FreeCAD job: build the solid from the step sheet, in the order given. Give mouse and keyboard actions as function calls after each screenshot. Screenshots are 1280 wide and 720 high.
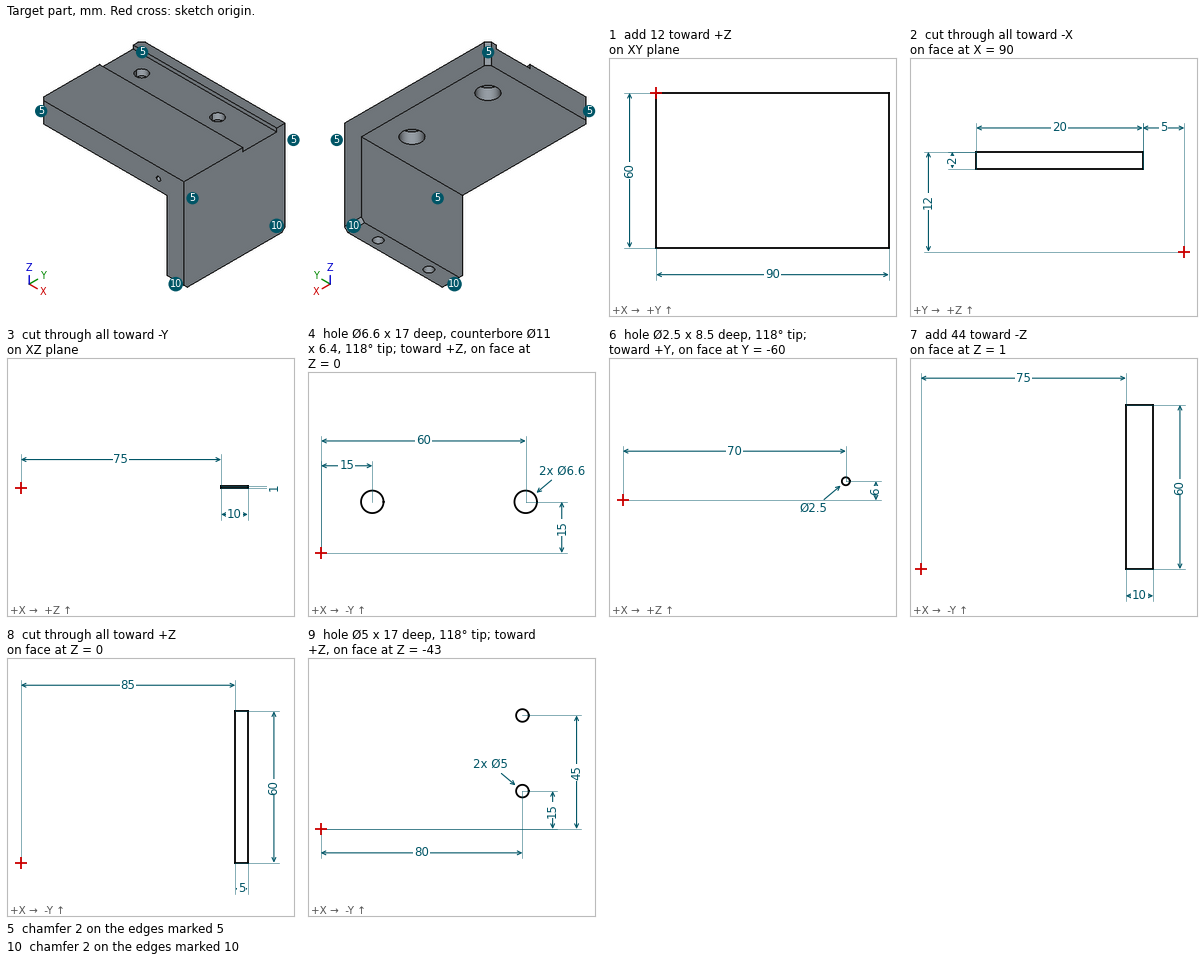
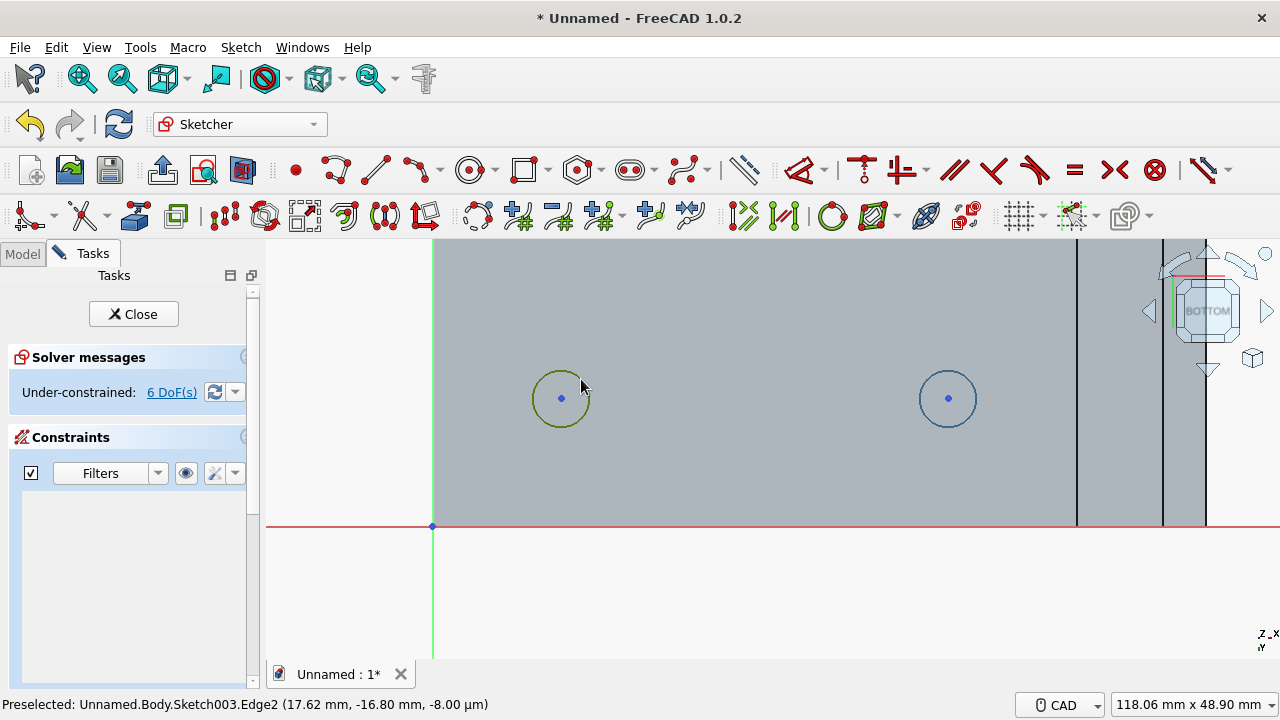
key(e)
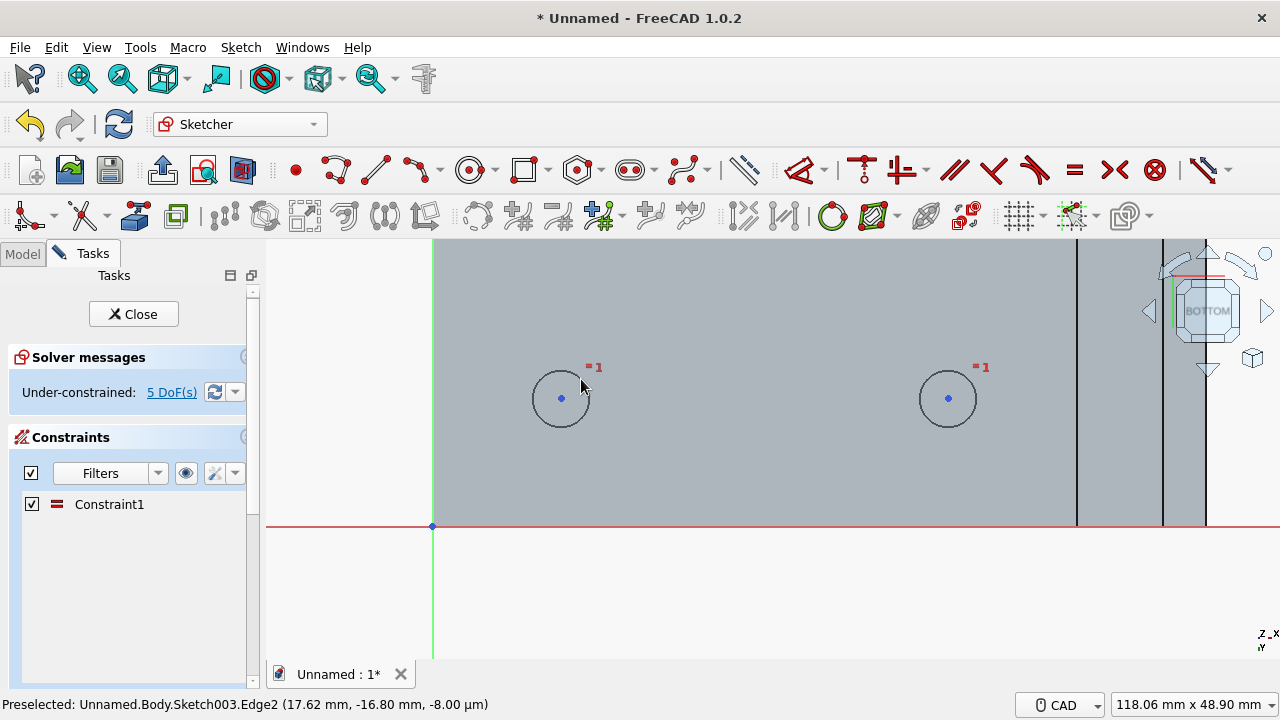
click(948, 399)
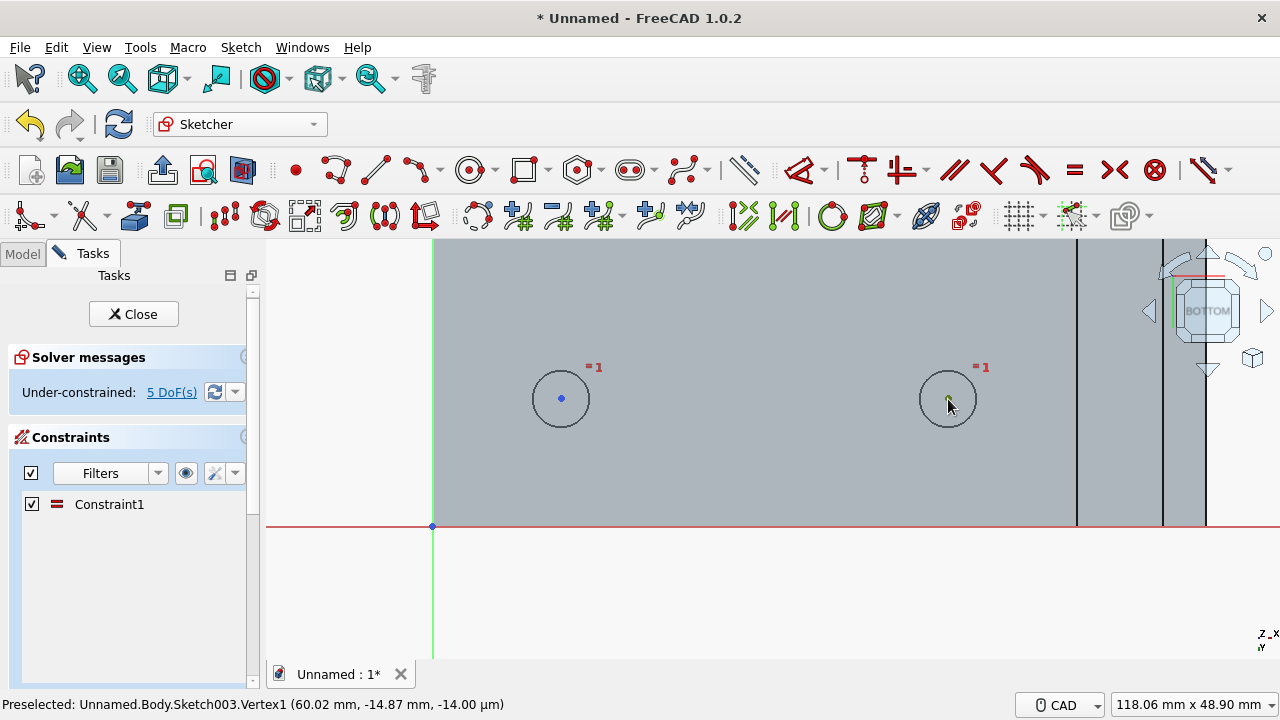
click(561, 399)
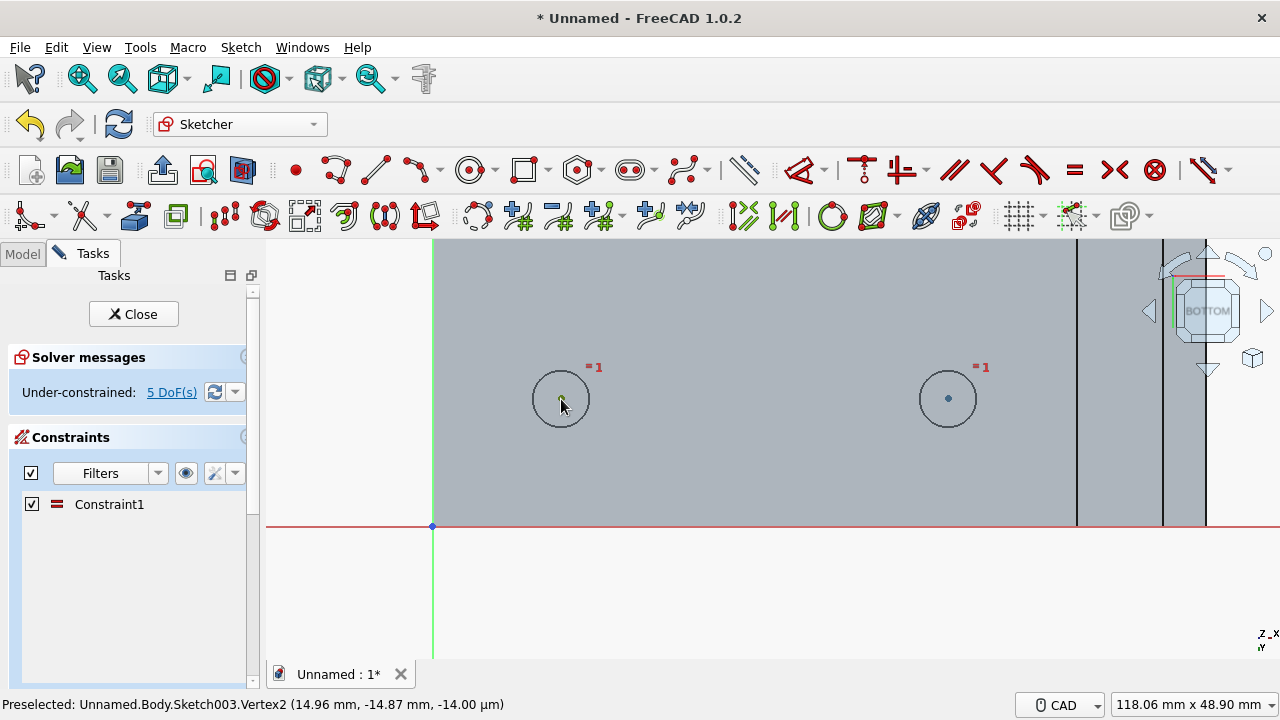
key(h)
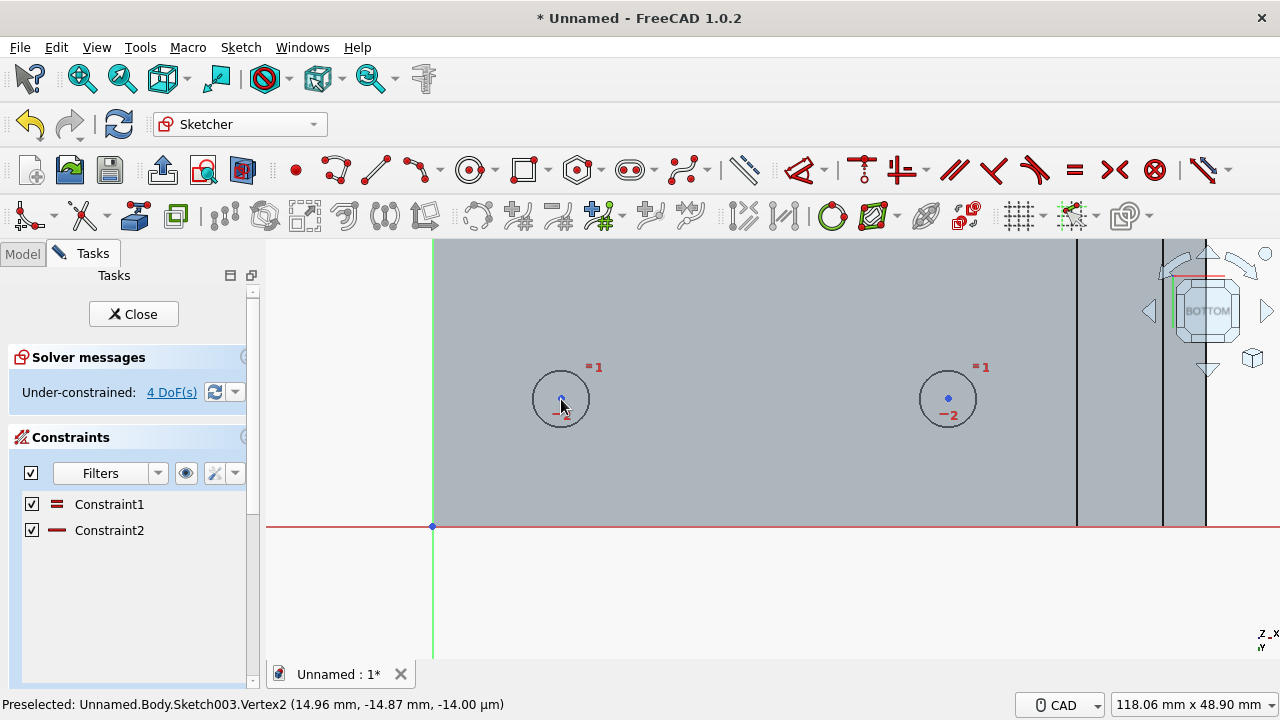
key(d)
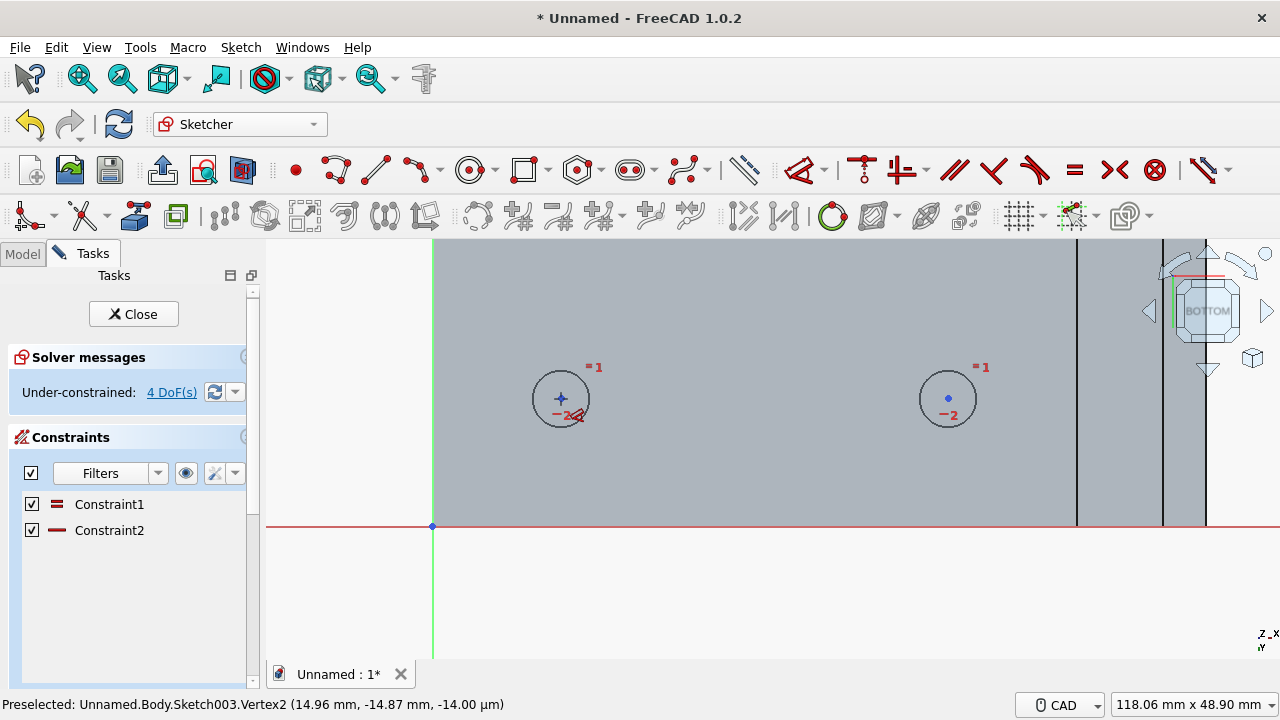
click(968, 379)
click(991, 356)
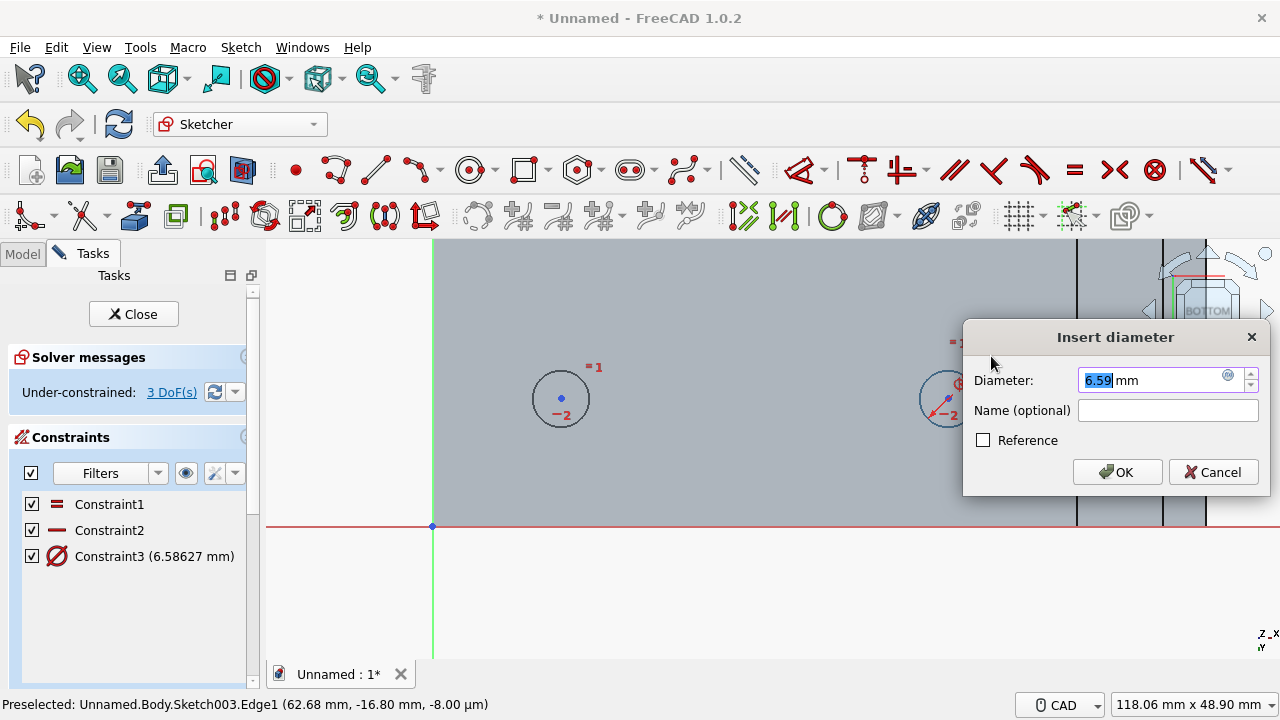
text(6.6)
key(Return)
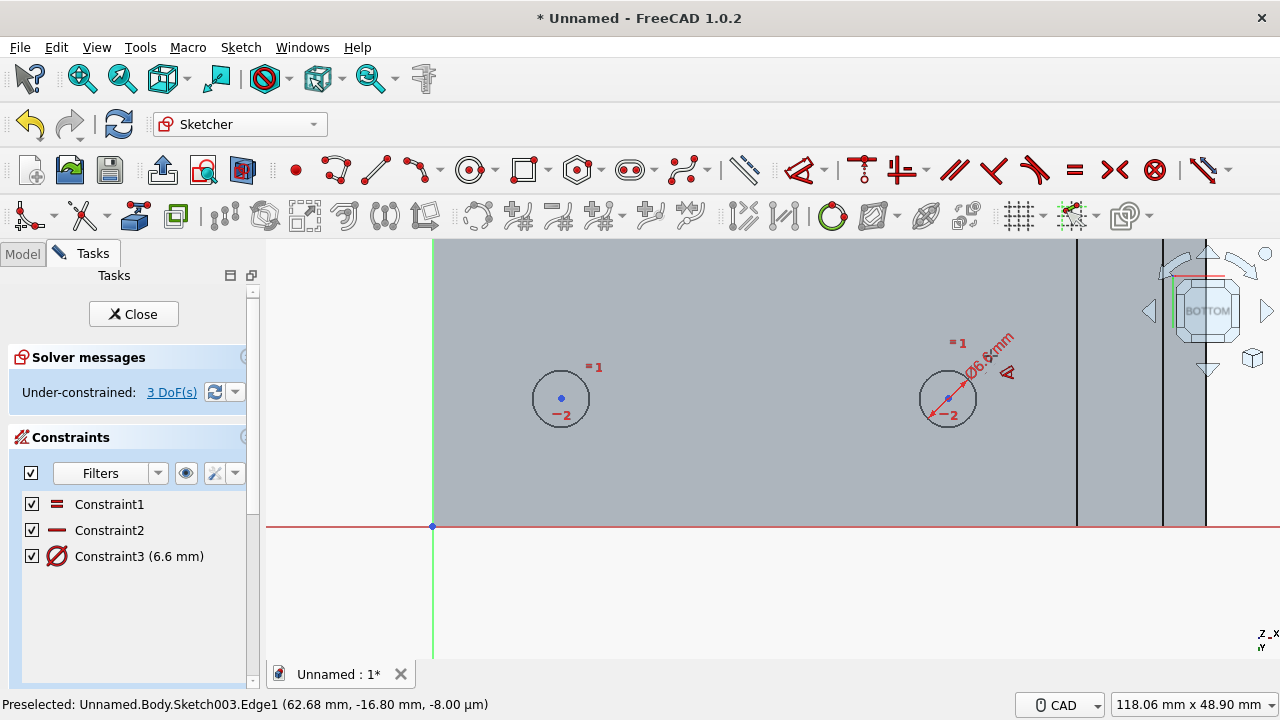
click(948, 399)
click(690, 561)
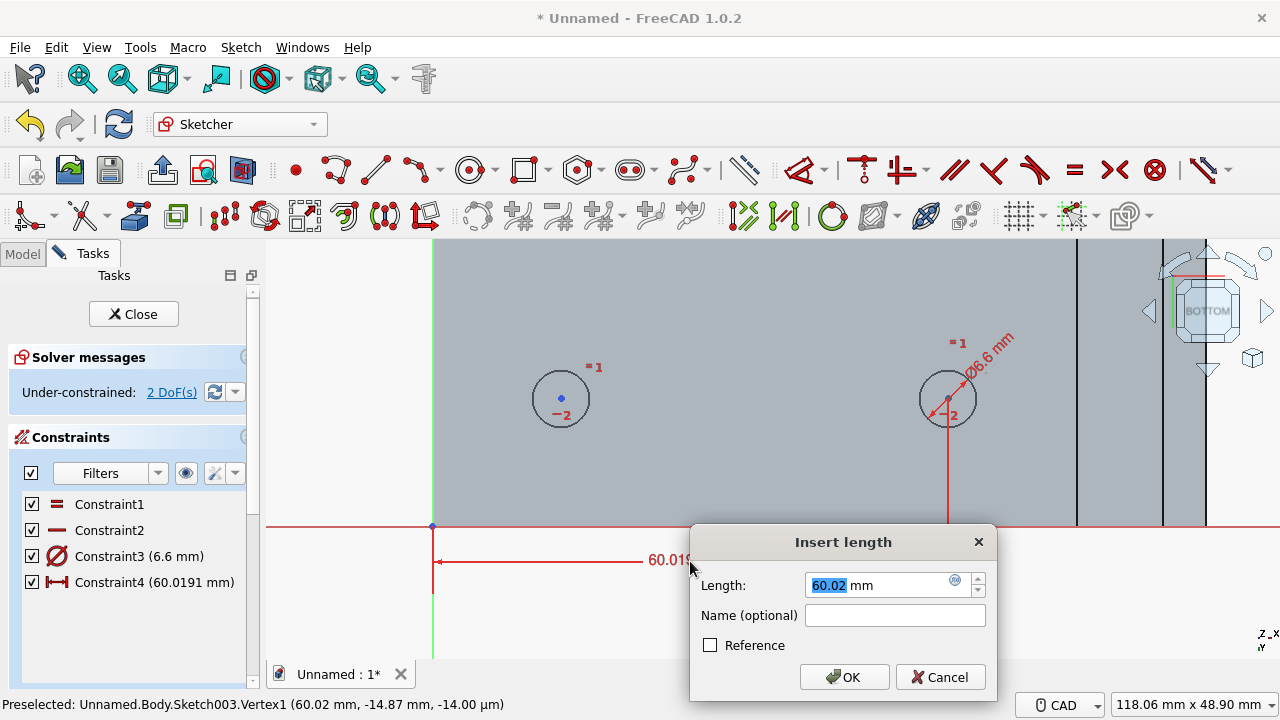
text(60)
key(Return)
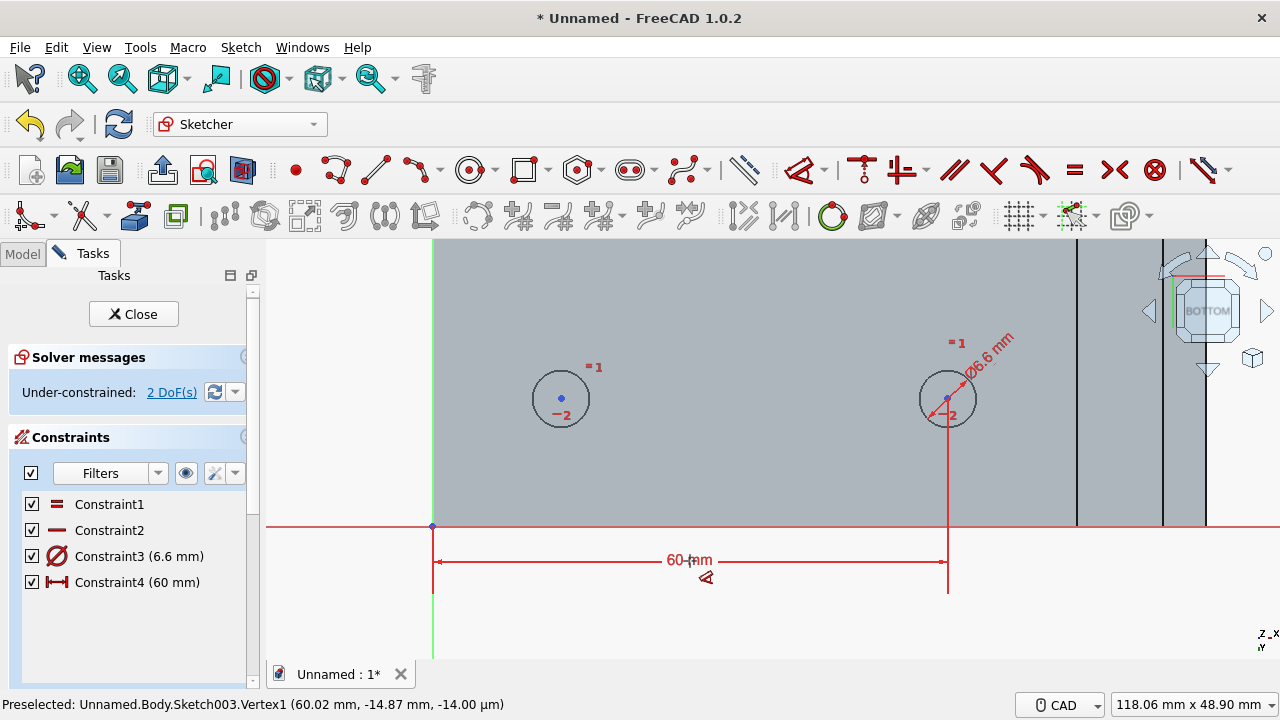
click(948, 399)
click(399, 463)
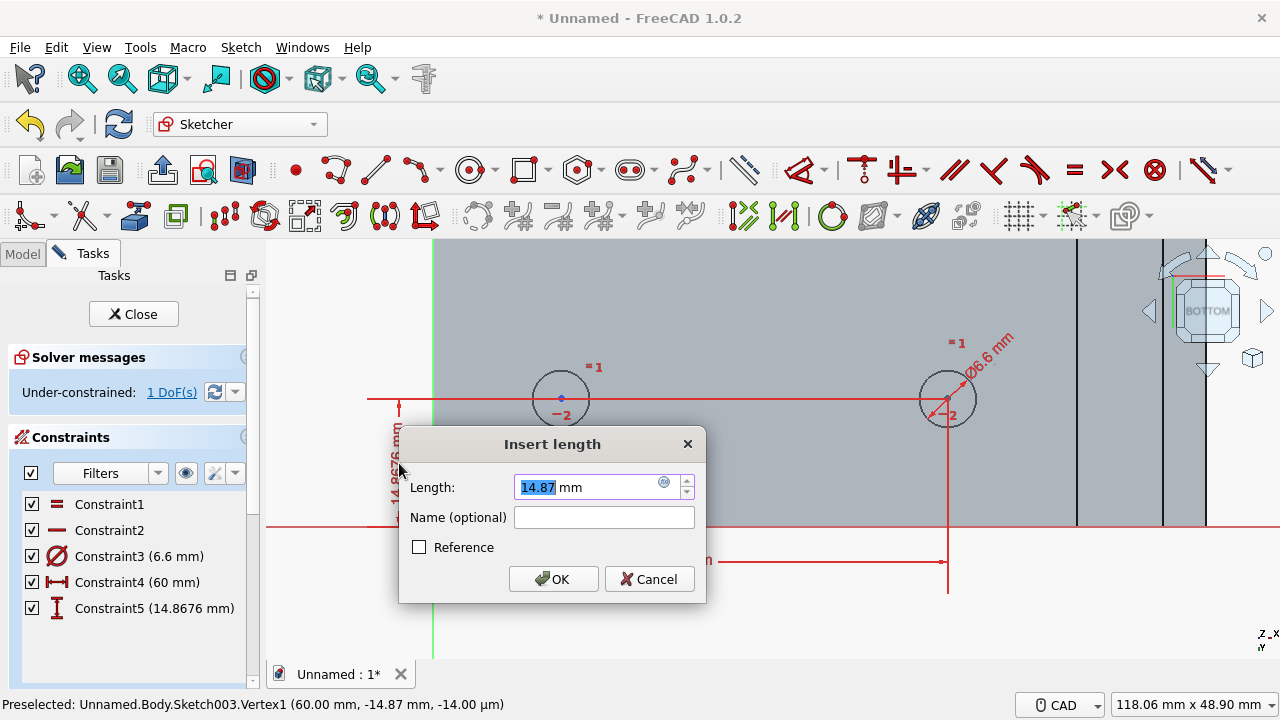
text(15)
key(Return)